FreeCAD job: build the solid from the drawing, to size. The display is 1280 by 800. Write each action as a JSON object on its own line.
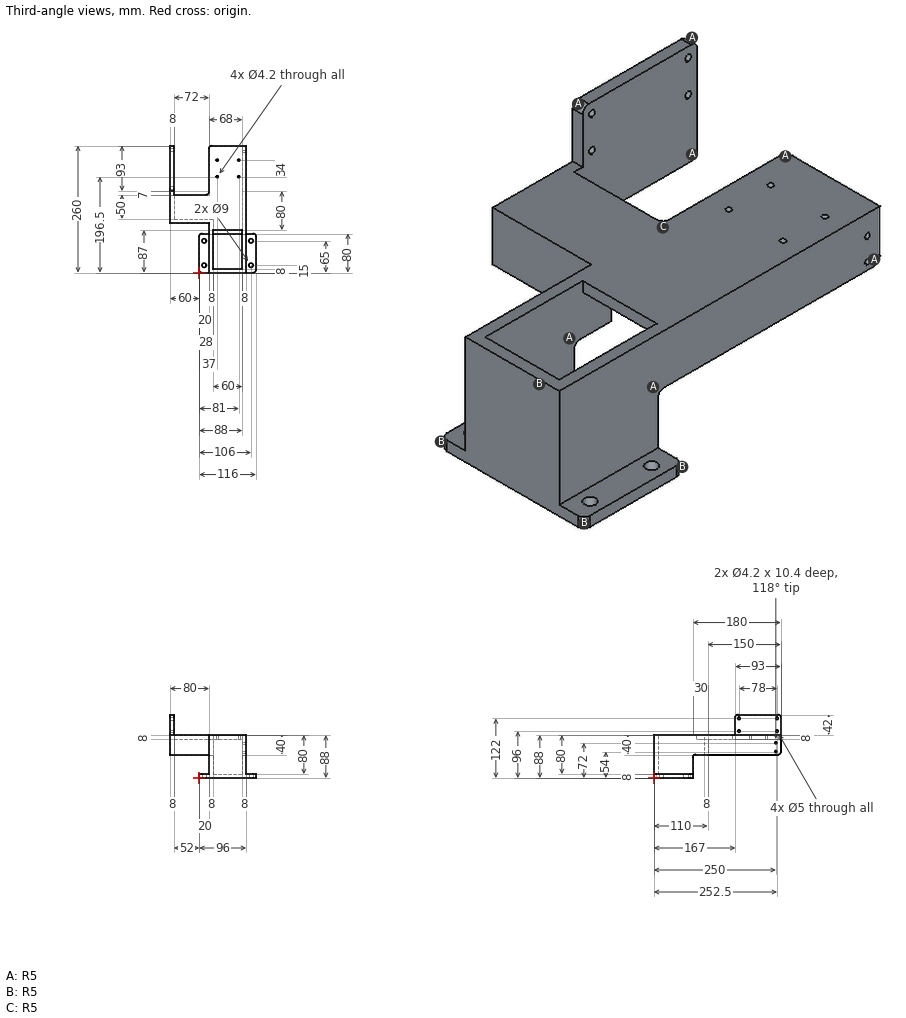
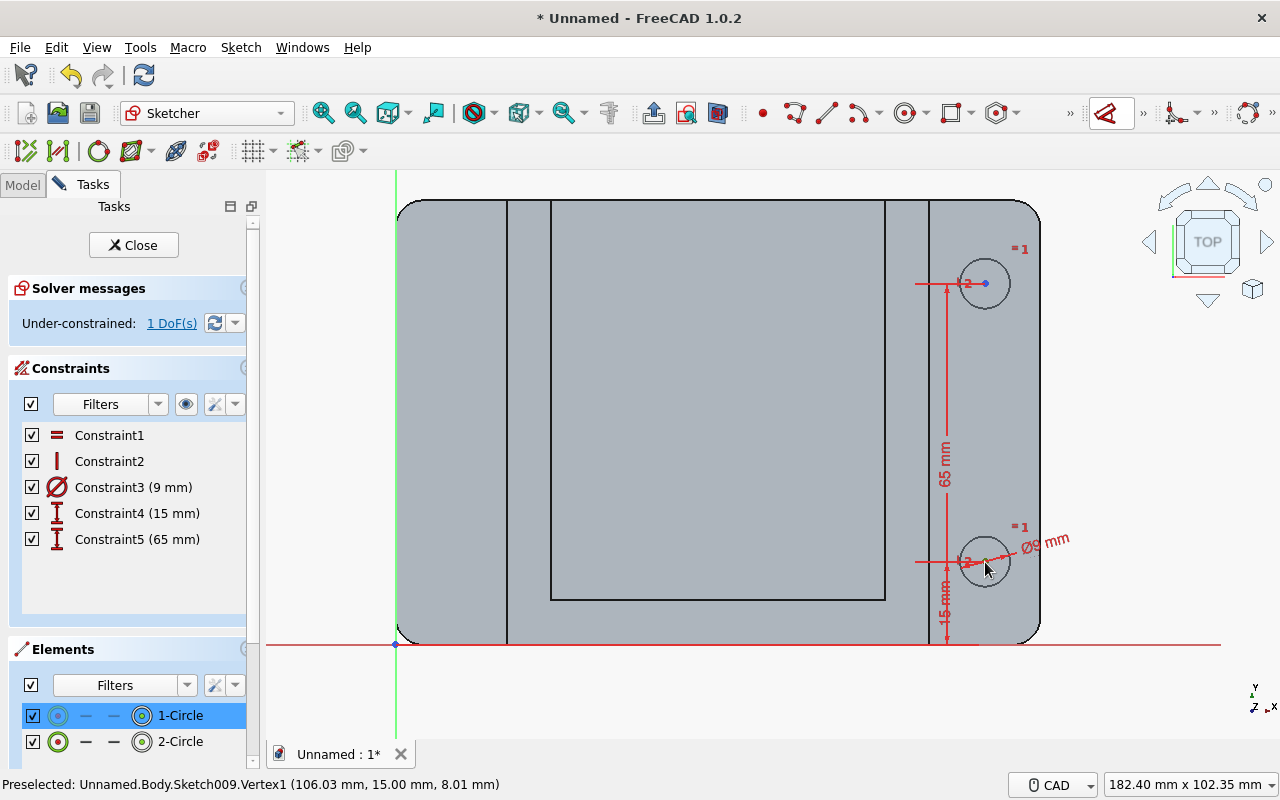
{"action": "key", "text": "l"}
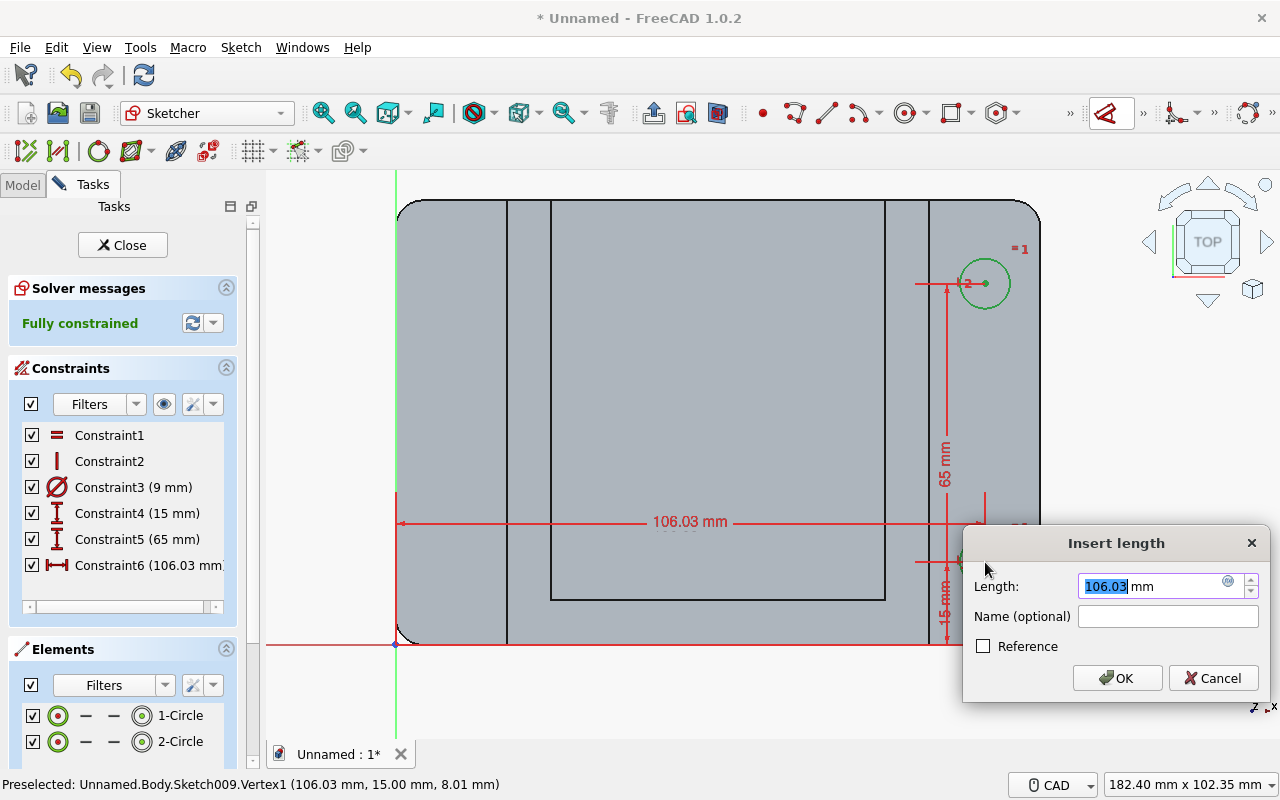
{"action": "type", "text": "106"}
{"action": "key", "text": "Return"}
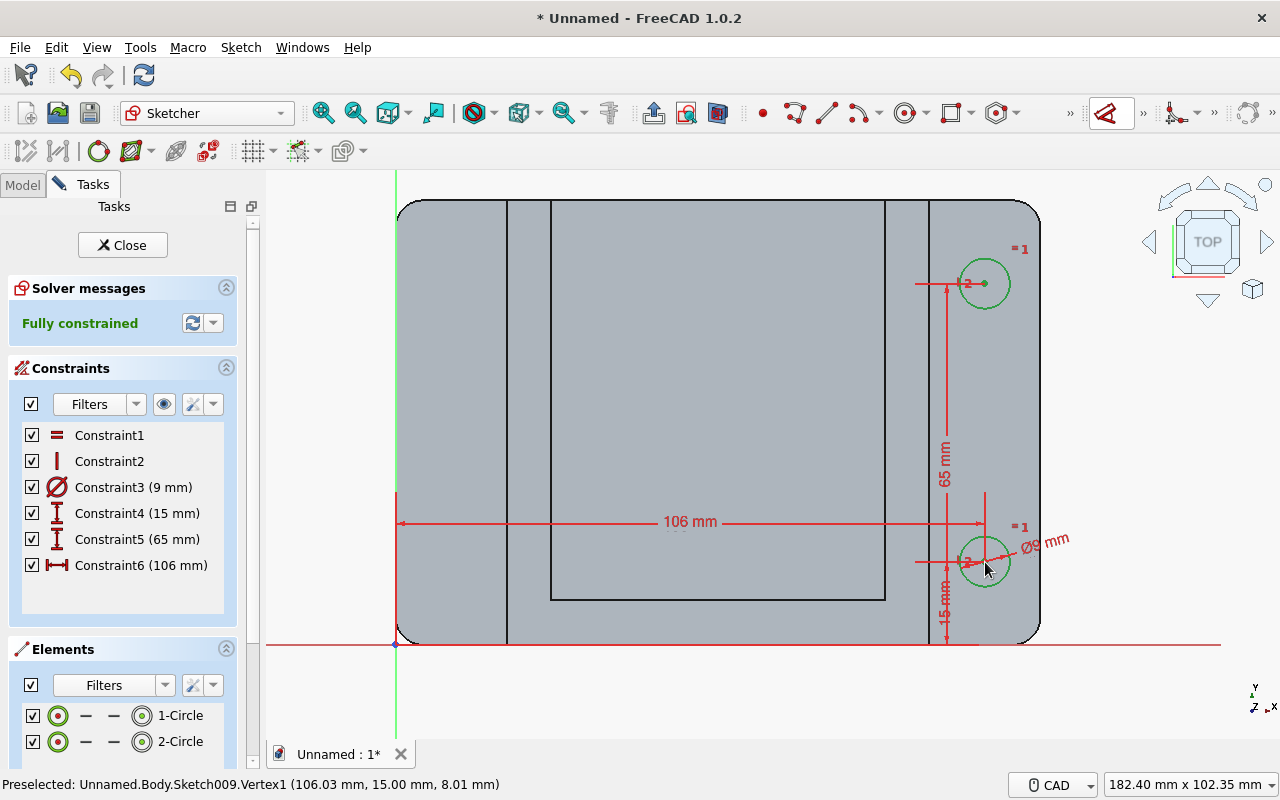
{"action": "left_click", "coordinate": [123, 245]}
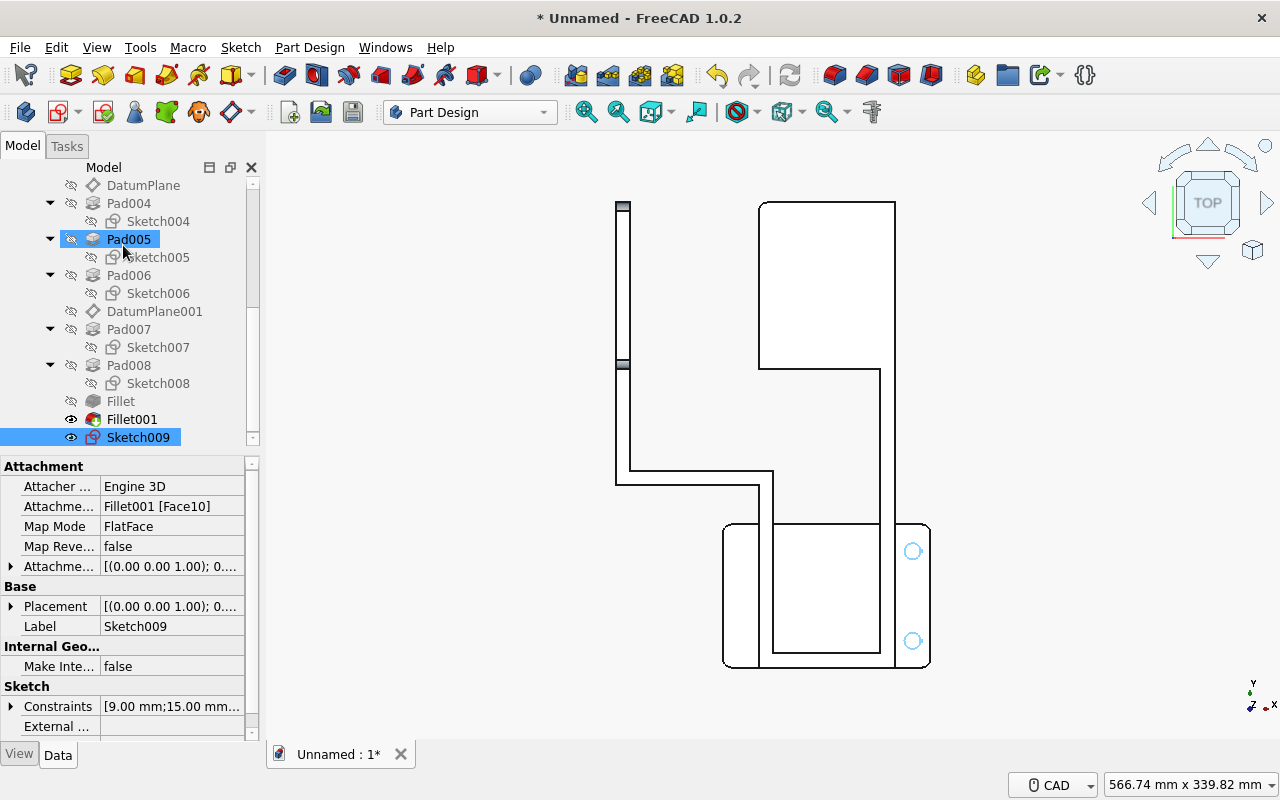
{"action": "left_click", "coordinate": [286, 76]}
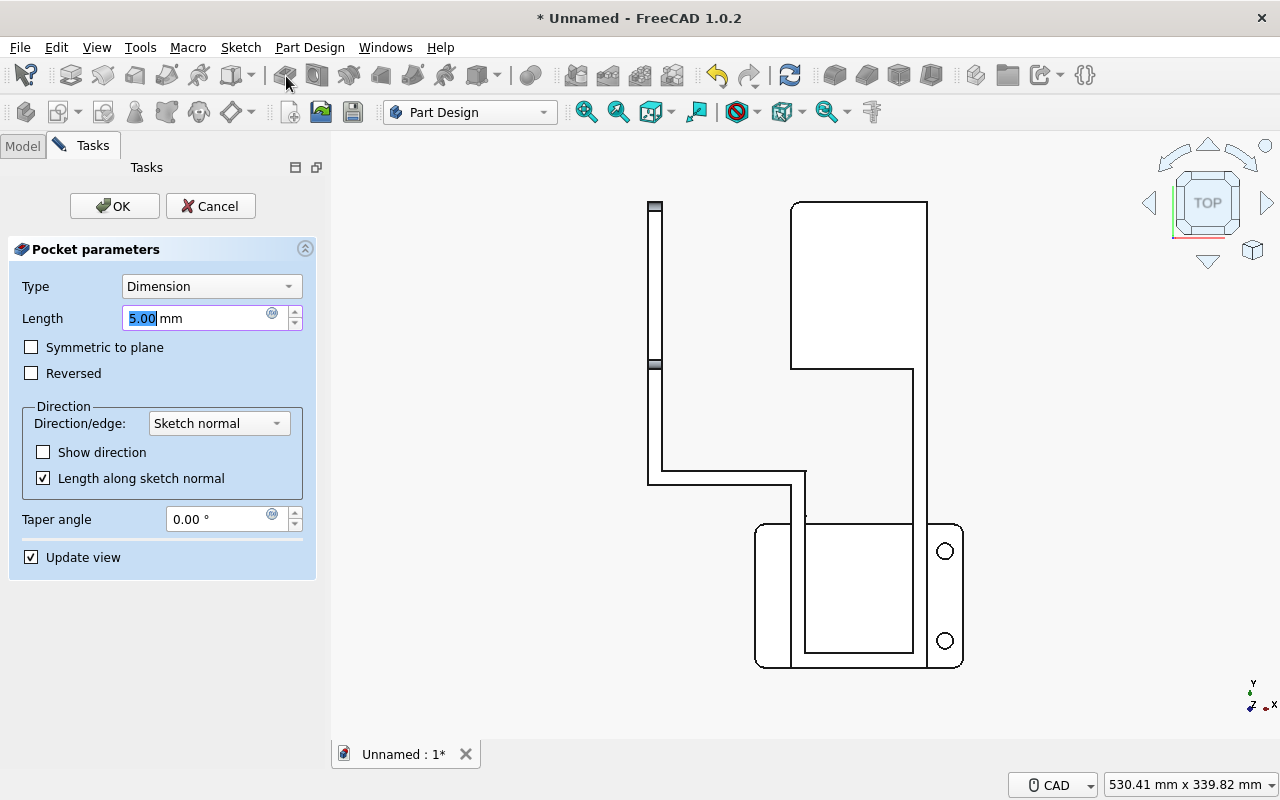
{"action": "left_click", "coordinate": [212, 286]}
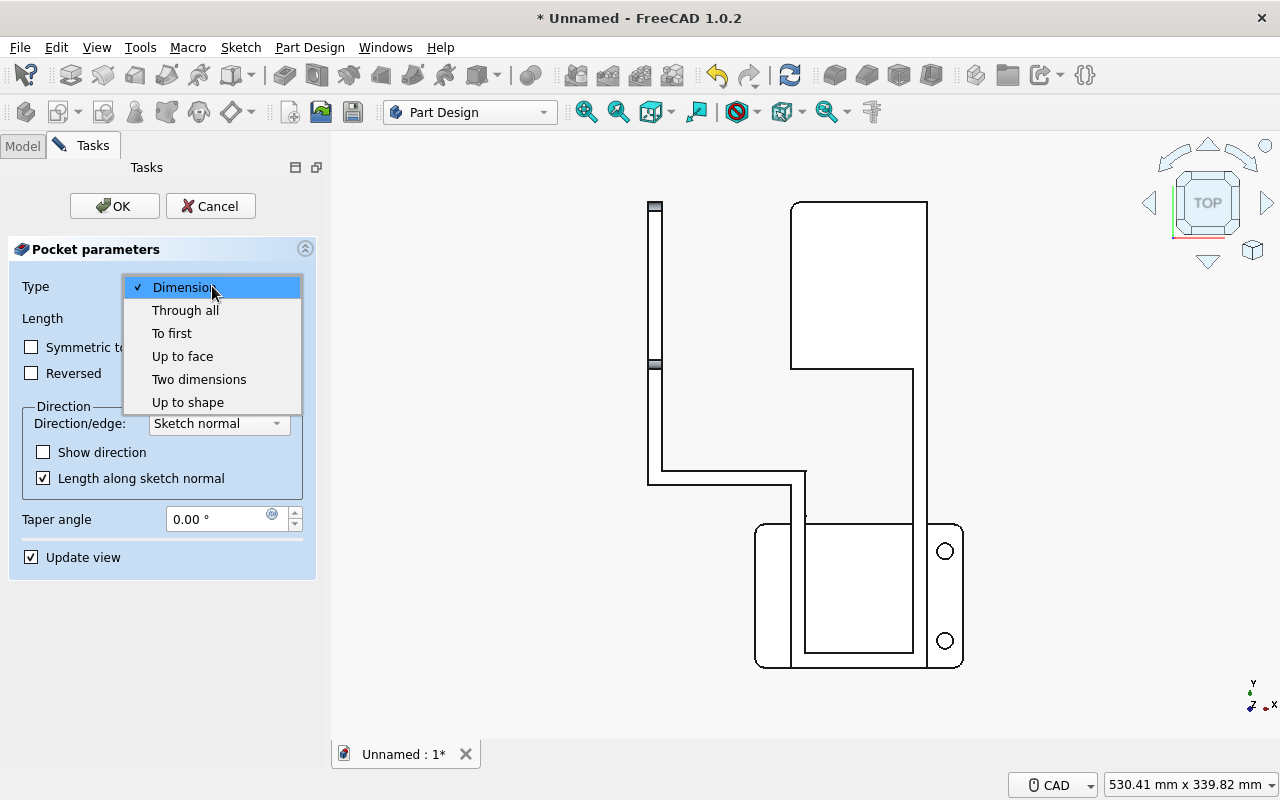
{"action": "left_click", "coordinate": [212, 310]}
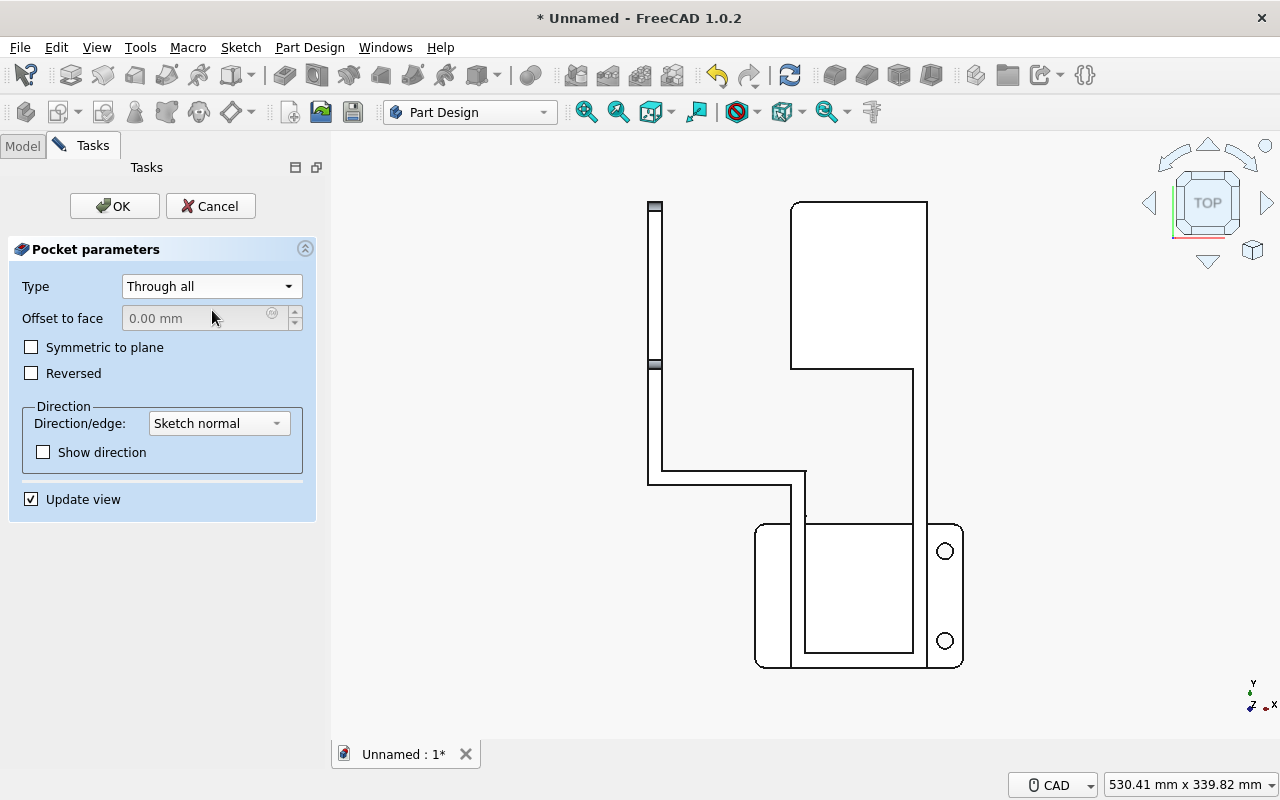
{"action": "left_click", "coordinate": [115, 206]}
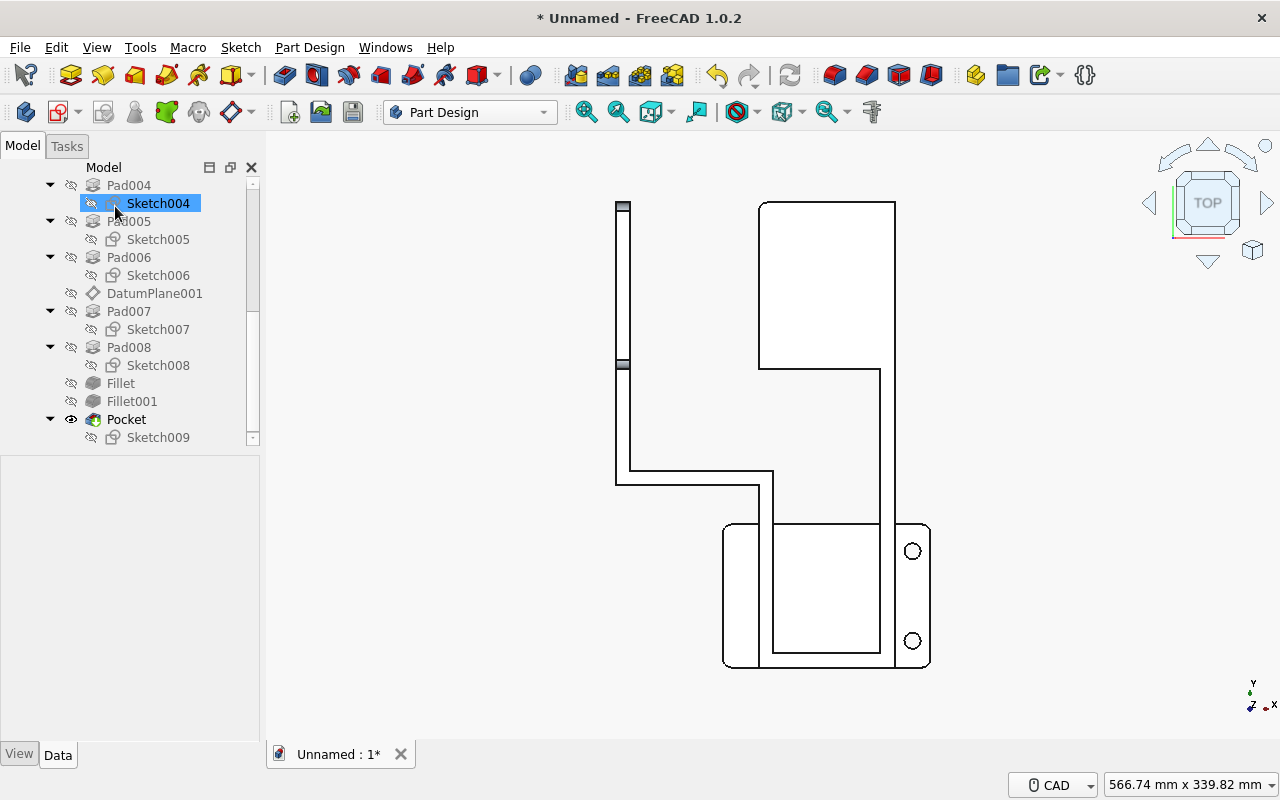
{"action": "scroll", "coordinate": [140, 307], "scroll_direction": "down", "scroll_amount": 3}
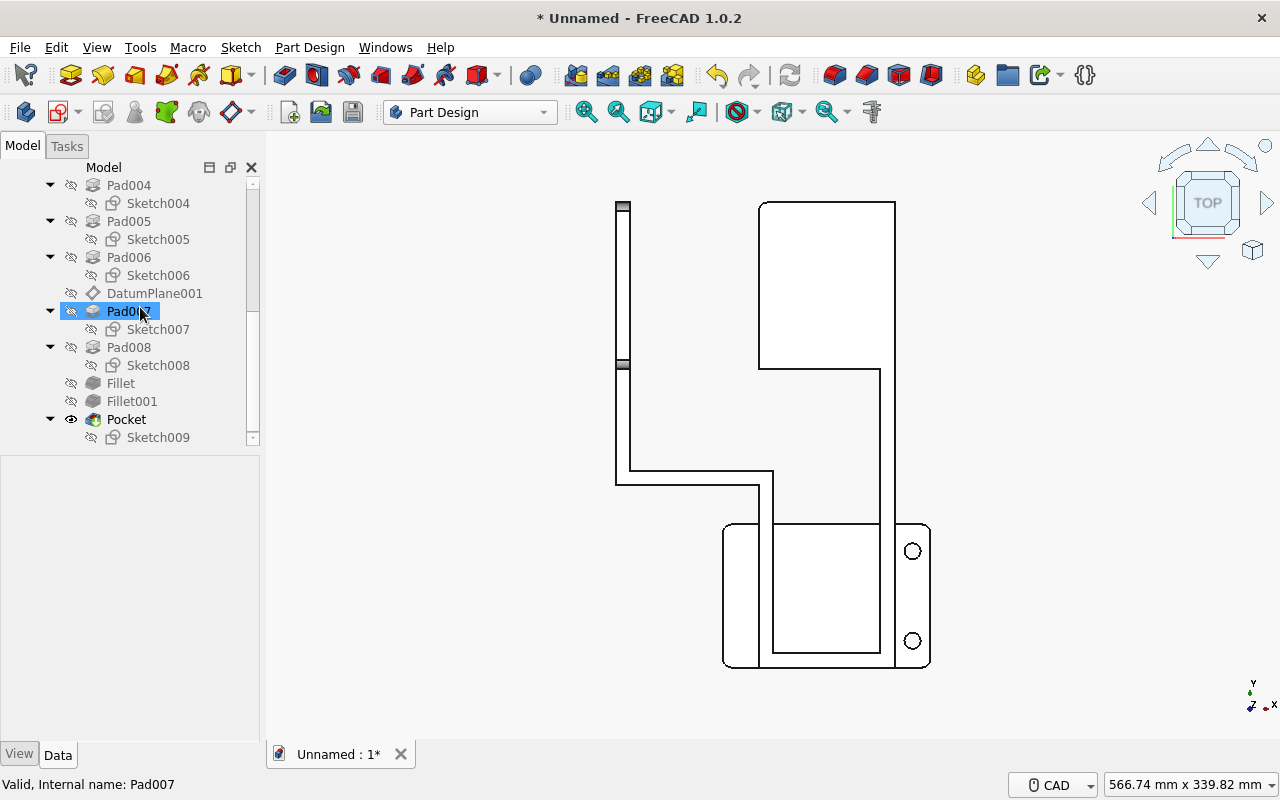
{"action": "scroll", "coordinate": [140, 307], "scroll_direction": "up", "scroll_amount": 15}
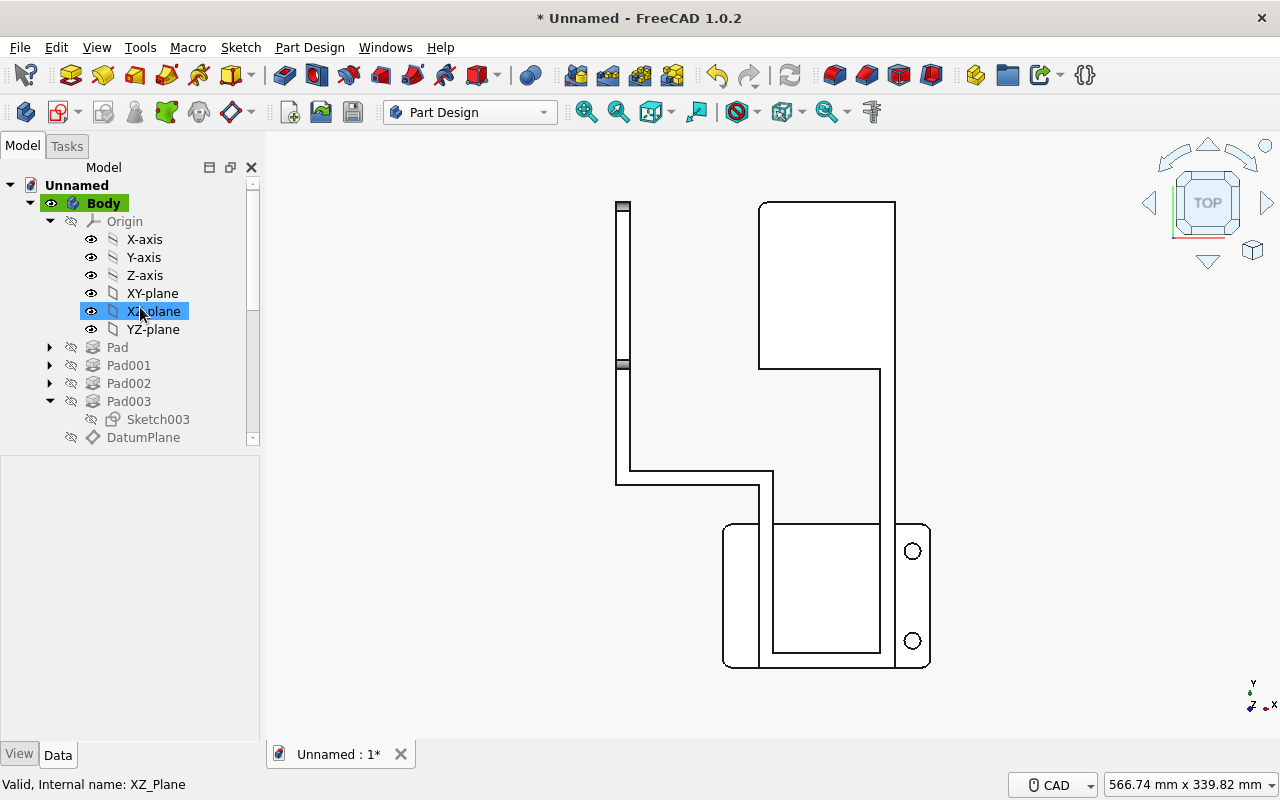
{"action": "left_click", "coordinate": [136, 329]}